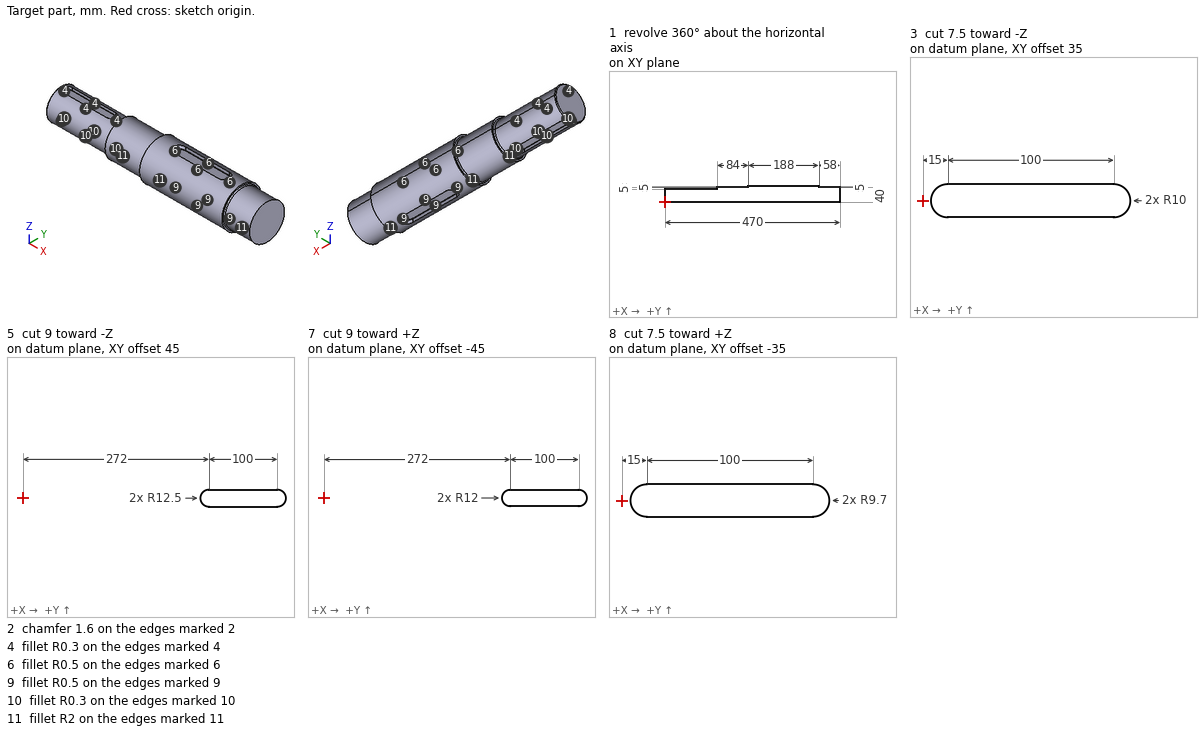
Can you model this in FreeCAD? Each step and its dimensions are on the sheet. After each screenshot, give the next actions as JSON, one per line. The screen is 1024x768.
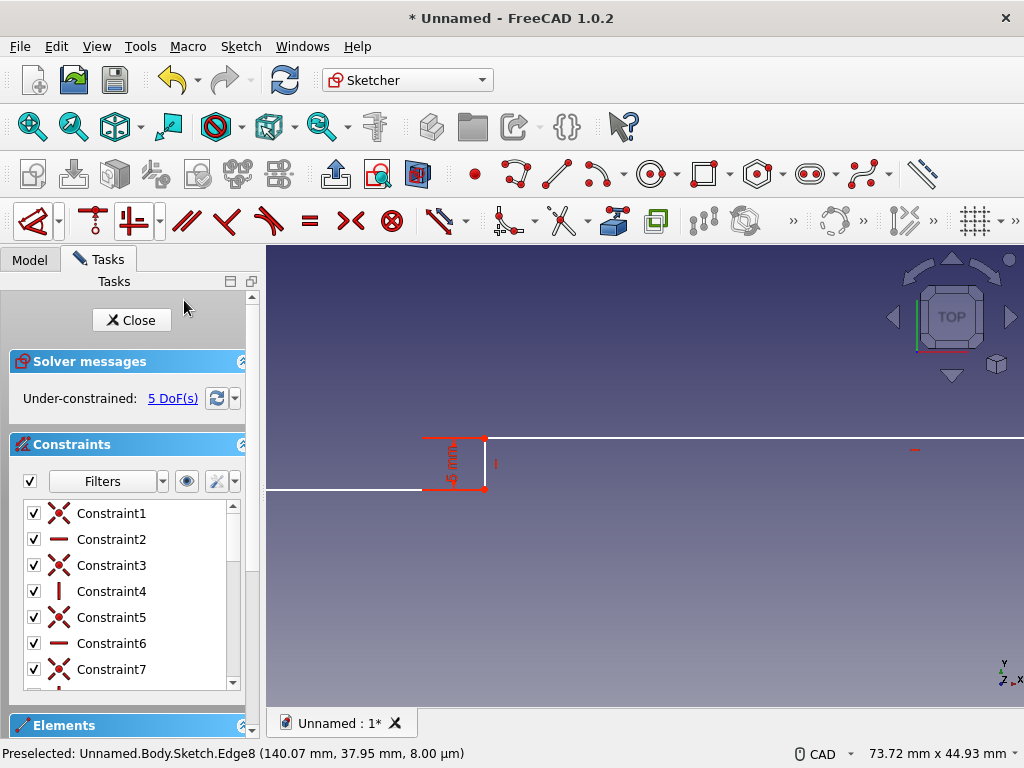
{"action": "scroll", "coordinate": [488, 462], "scroll_direction": "down", "scroll_amount": 12}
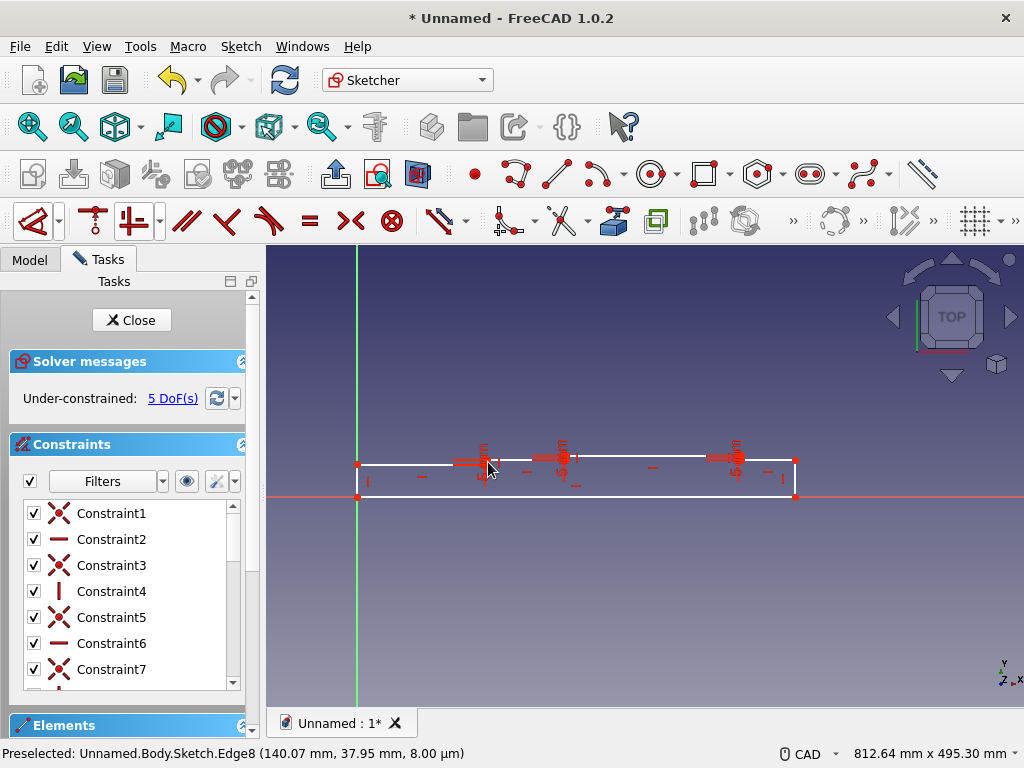
{"action": "scroll", "coordinate": [795, 486], "scroll_direction": "up", "scroll_amount": 2}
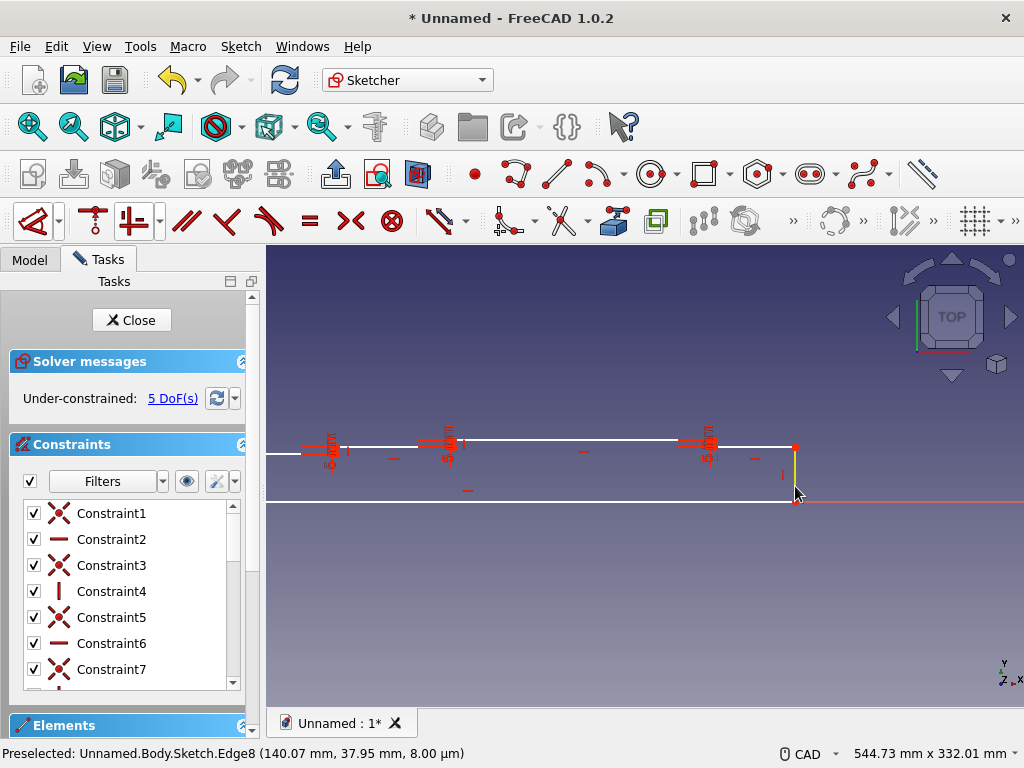
{"action": "left_click", "coordinate": [795, 486]}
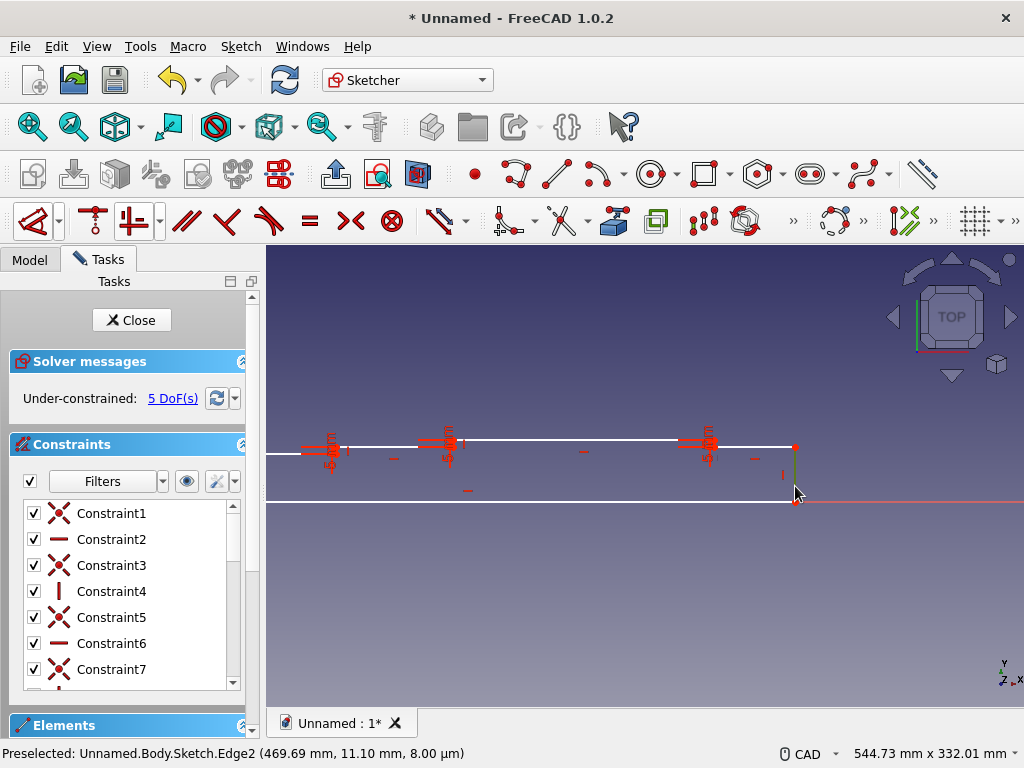
{"action": "left_click", "coordinate": [58, 222]}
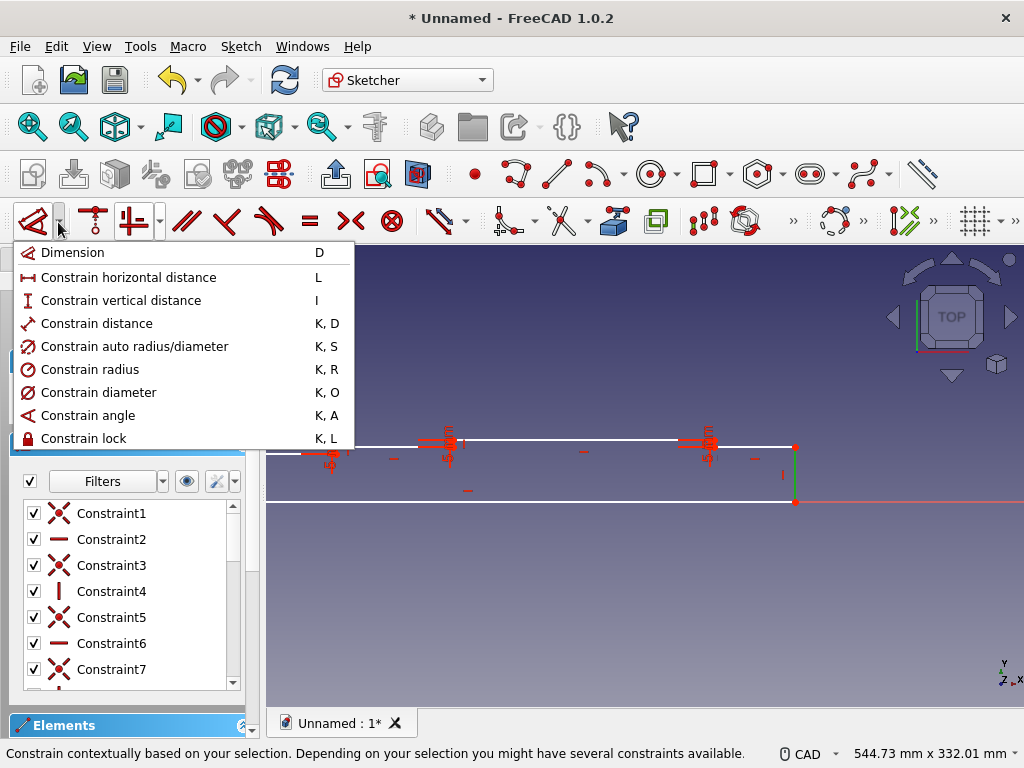
{"action": "left_click", "coordinate": [184, 300]}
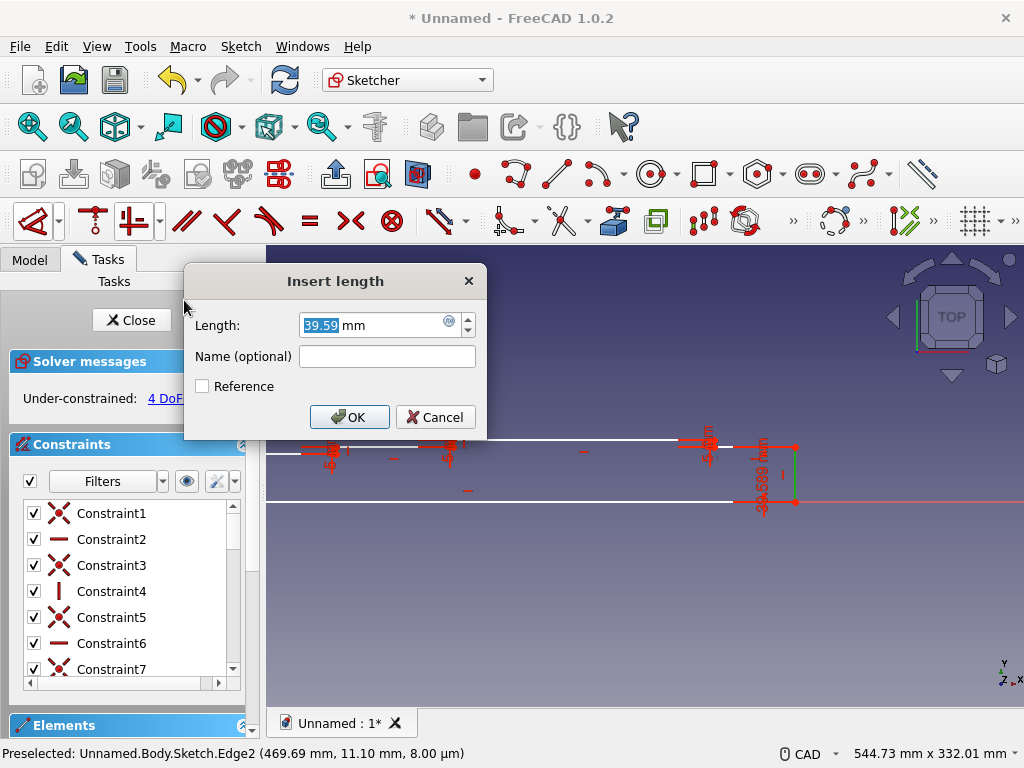
{"action": "type", "text": "40"}
{"action": "key", "text": "Return"}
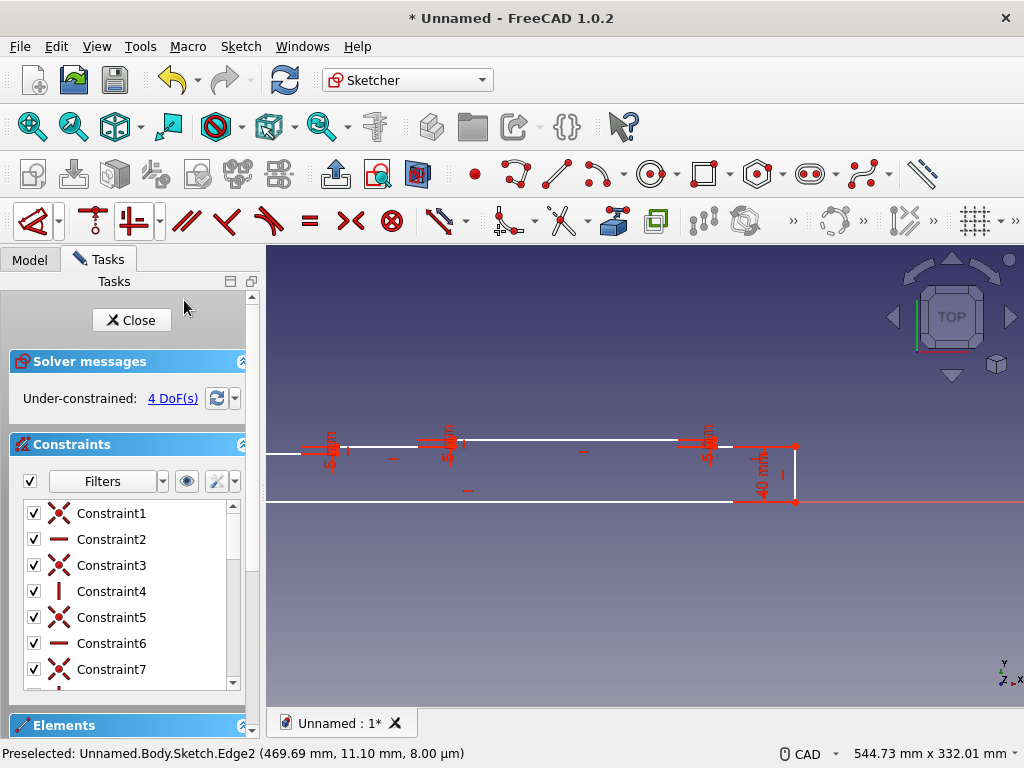
{"action": "left_click", "coordinate": [771, 447]}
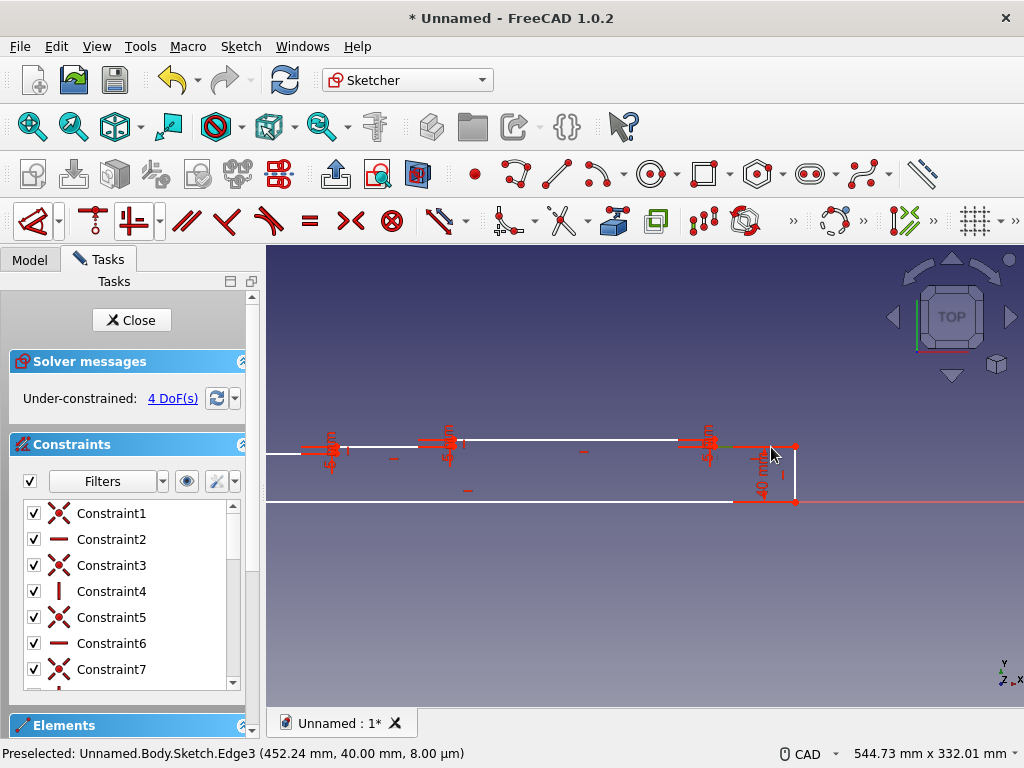
{"action": "left_click", "coordinate": [58, 222]}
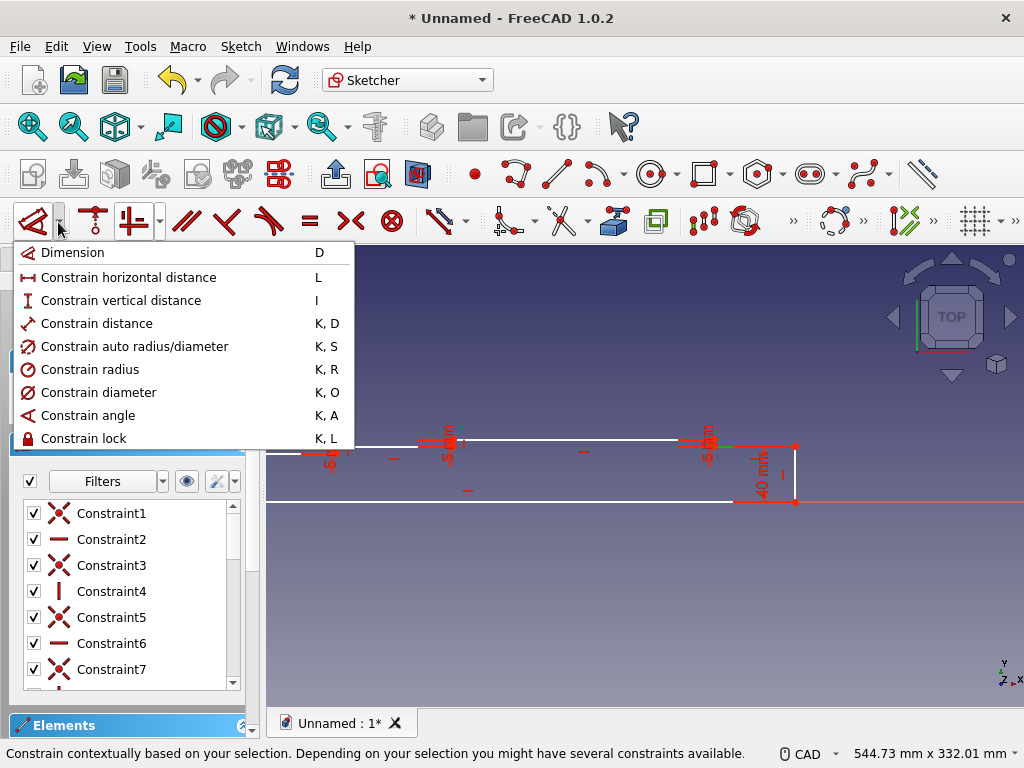
{"action": "left_click", "coordinate": [184, 278]}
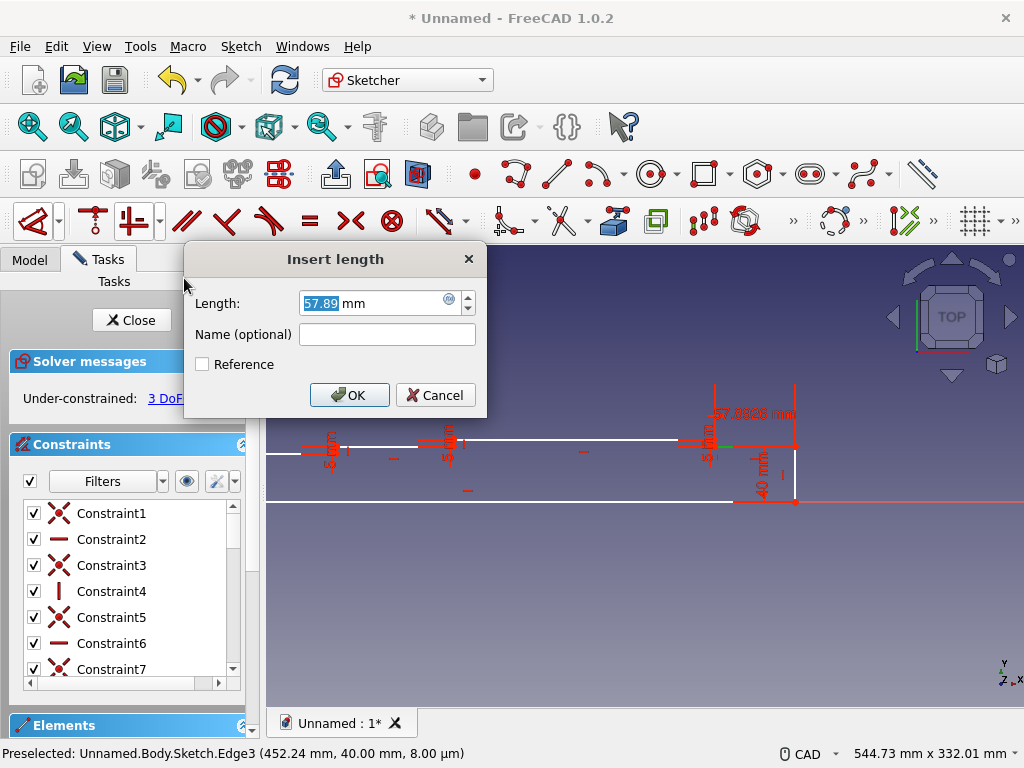
{"action": "type", "text": "58"}
{"action": "key", "text": "Return"}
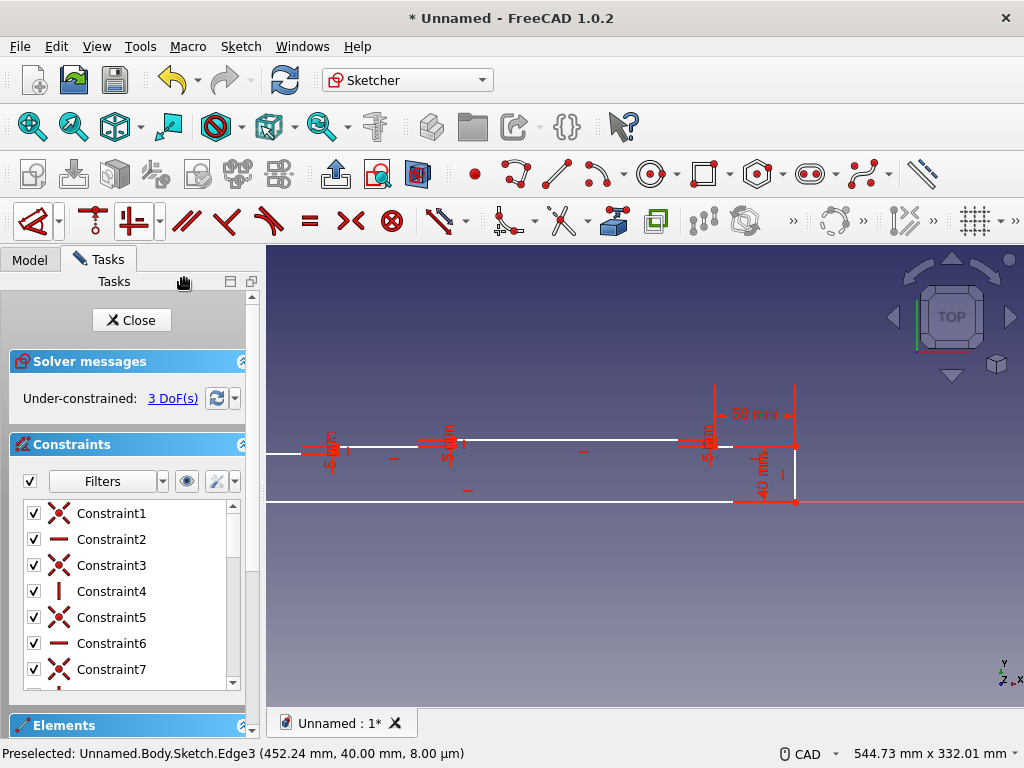
{"action": "left_click", "coordinate": [418, 447]}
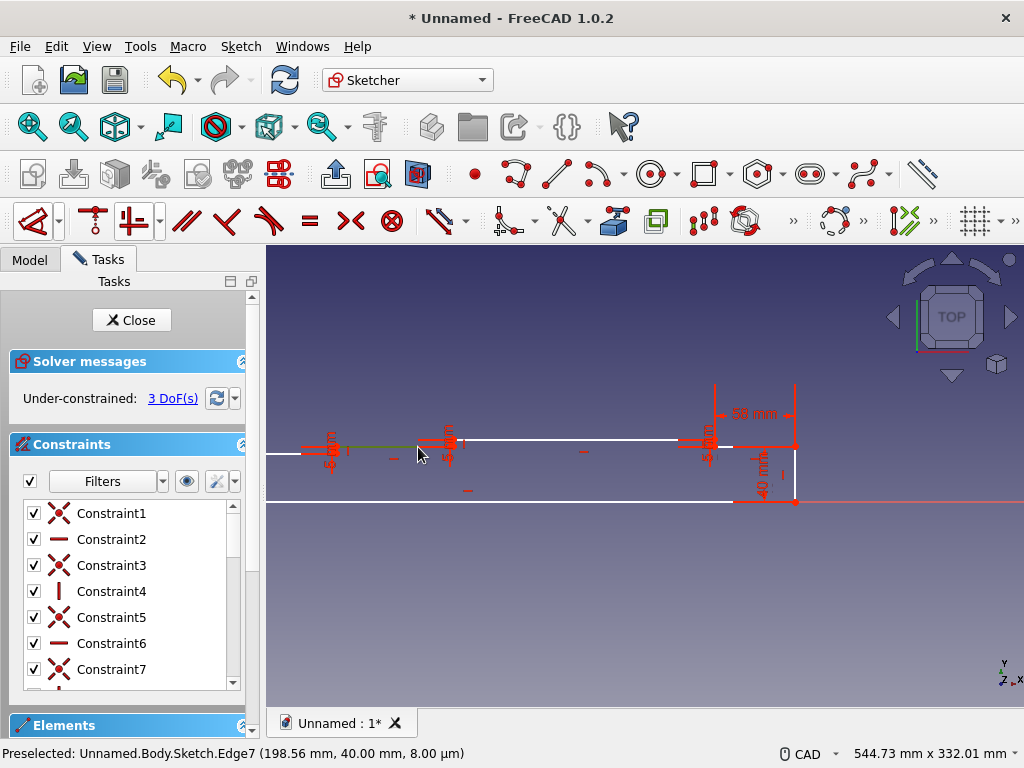
{"action": "key", "text": "l"}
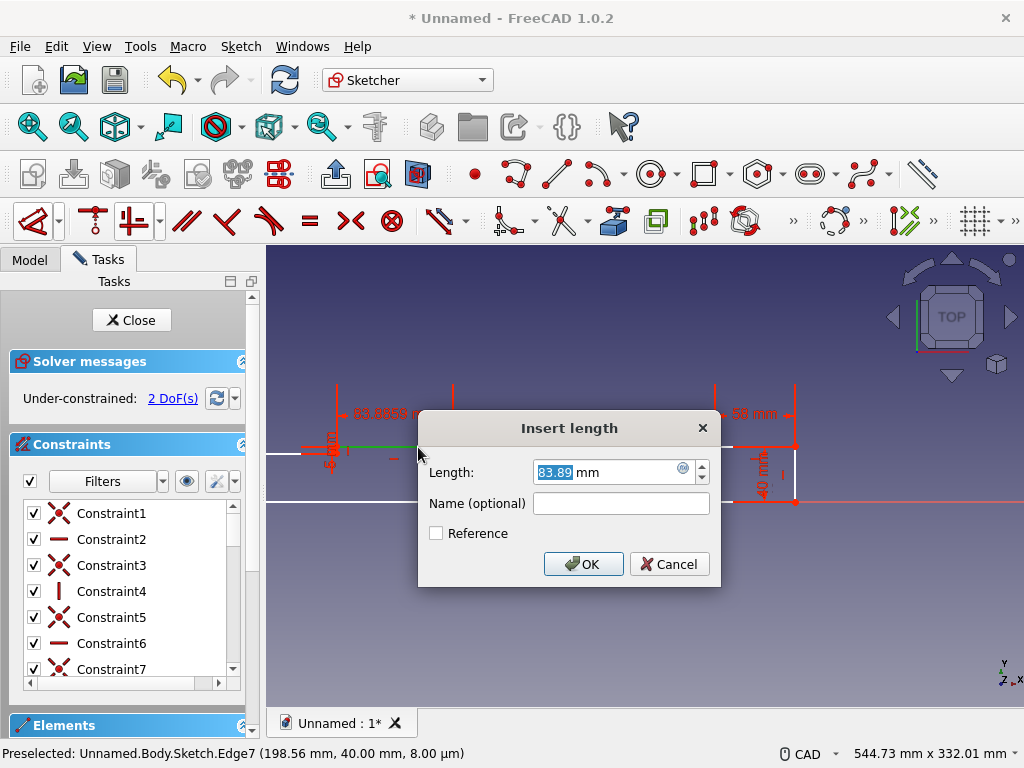
{"action": "type", "text": "84"}
{"action": "key", "text": "Return"}